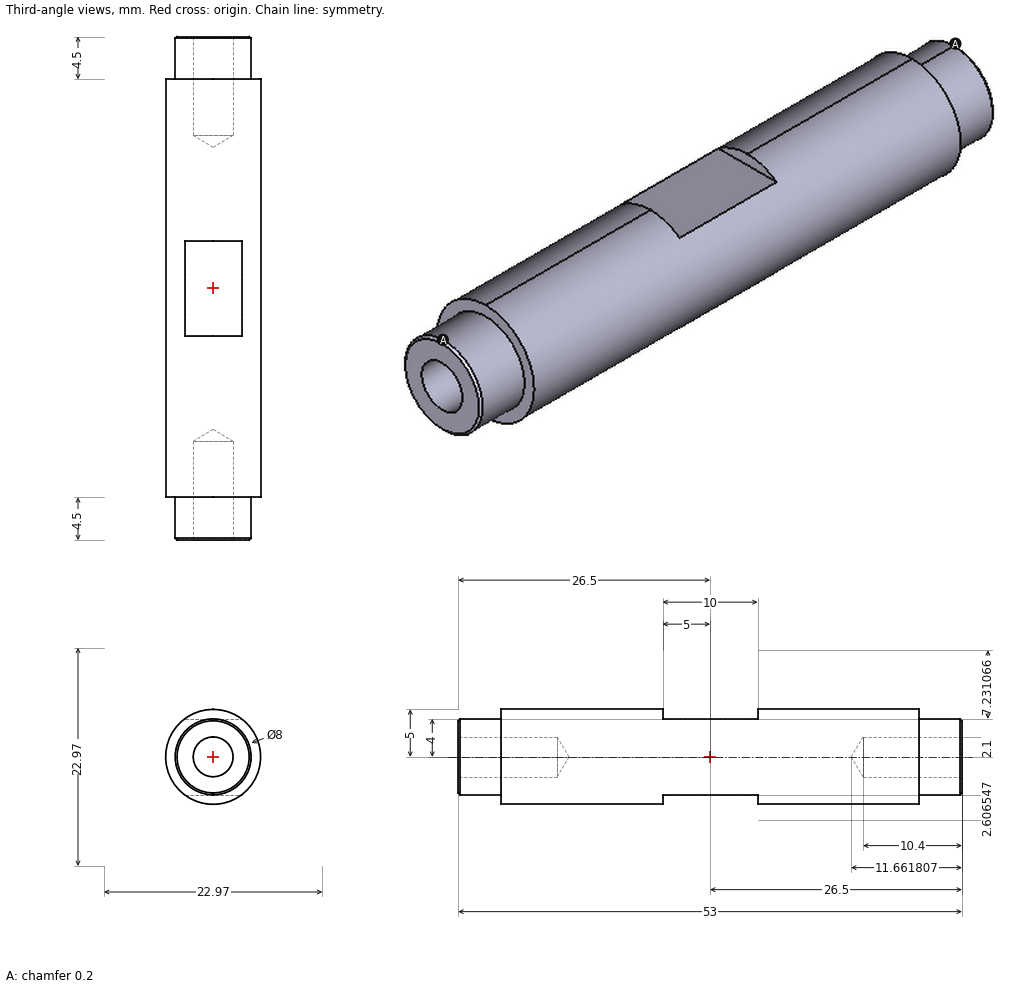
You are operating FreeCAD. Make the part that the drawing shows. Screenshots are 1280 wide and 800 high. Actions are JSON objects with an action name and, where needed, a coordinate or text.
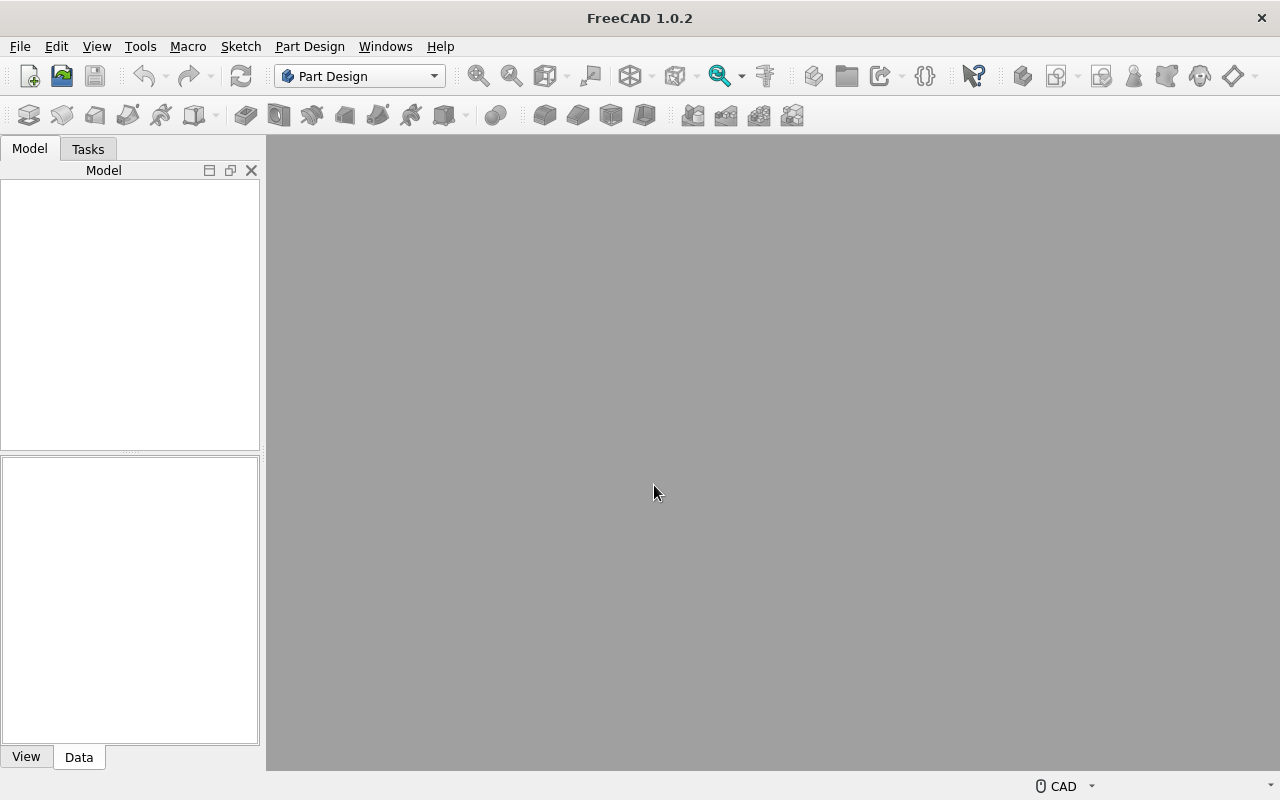
{"action": "left_click", "coordinate": [29, 76]}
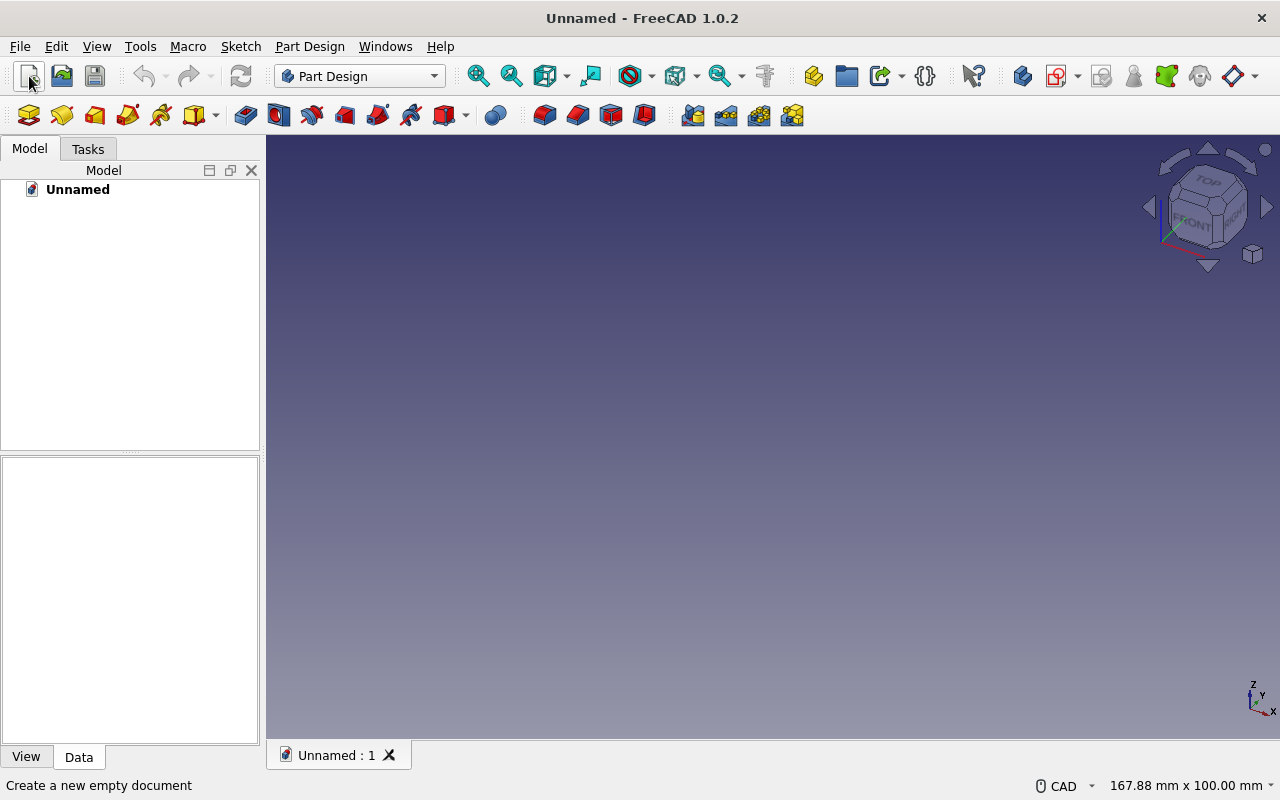
{"action": "left_click", "coordinate": [1056, 76]}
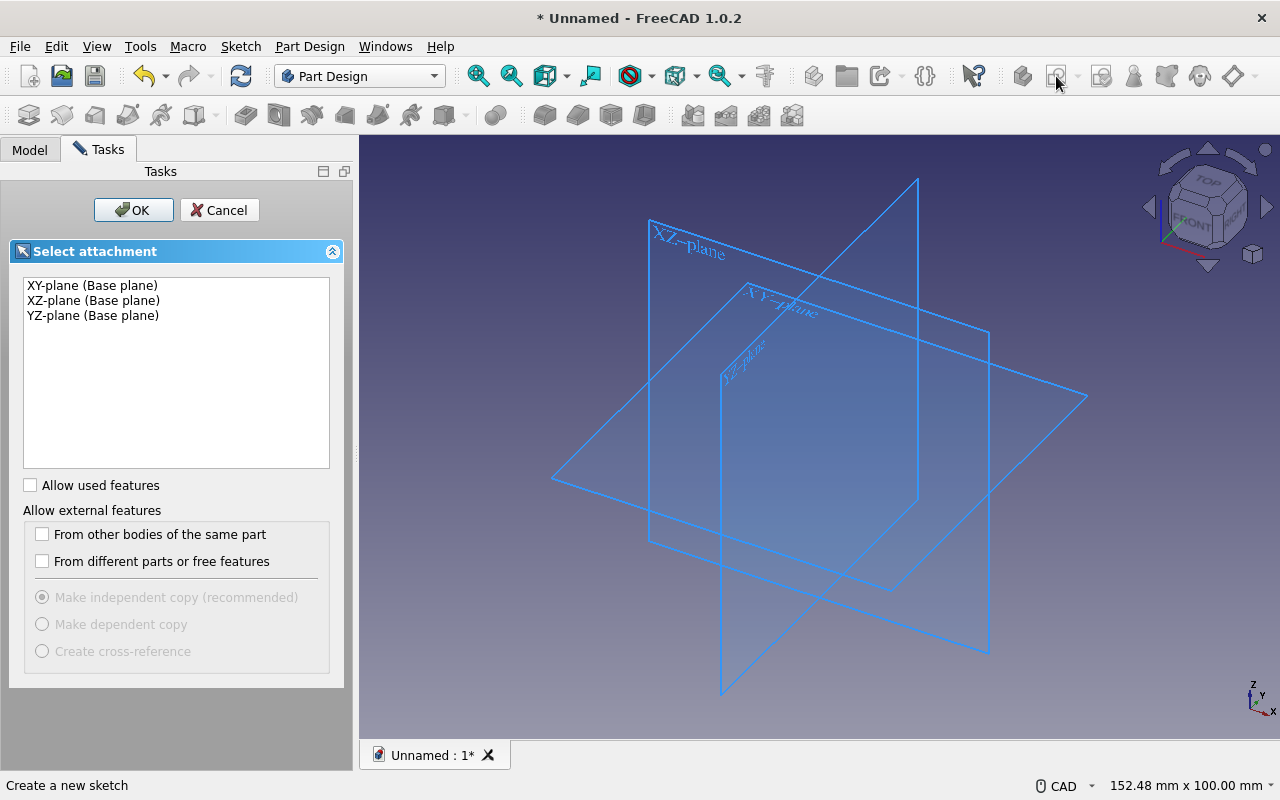
{"action": "left_click", "coordinate": [84, 316]}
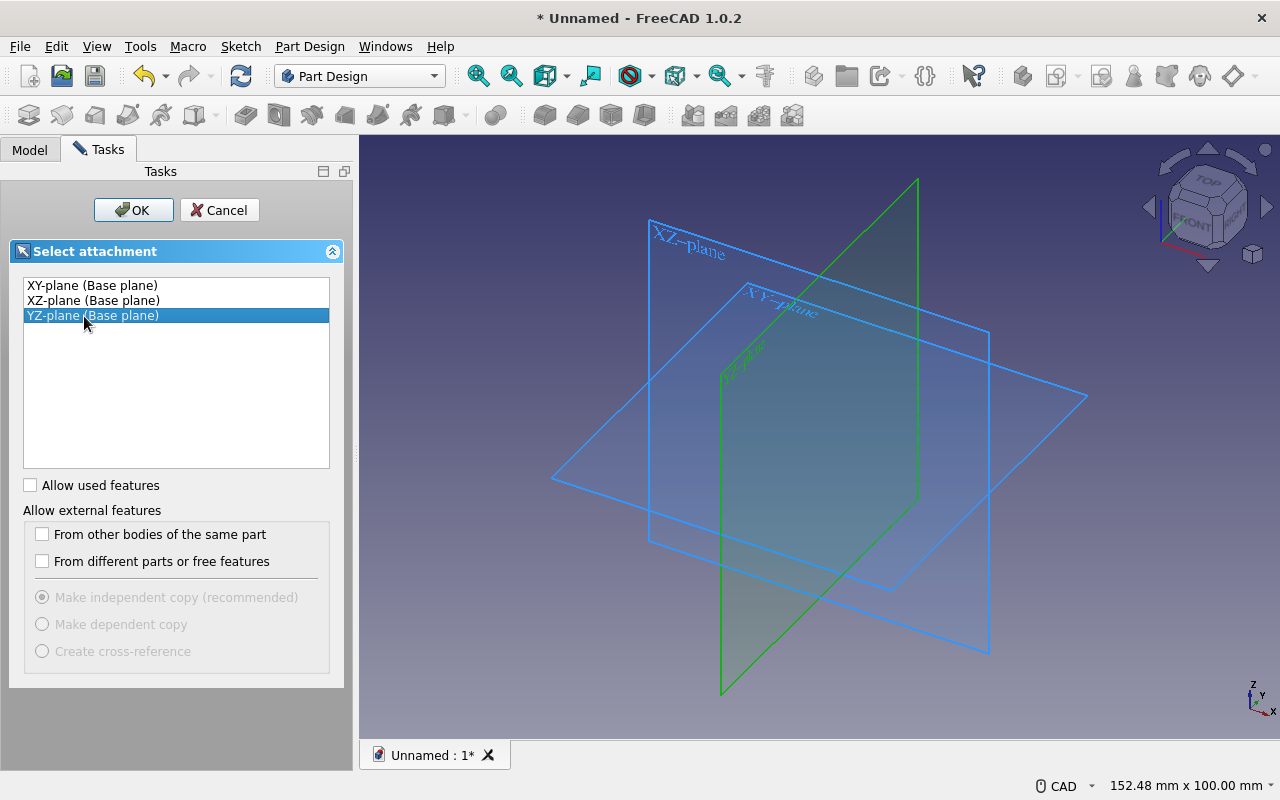
{"action": "left_click", "coordinate": [134, 210]}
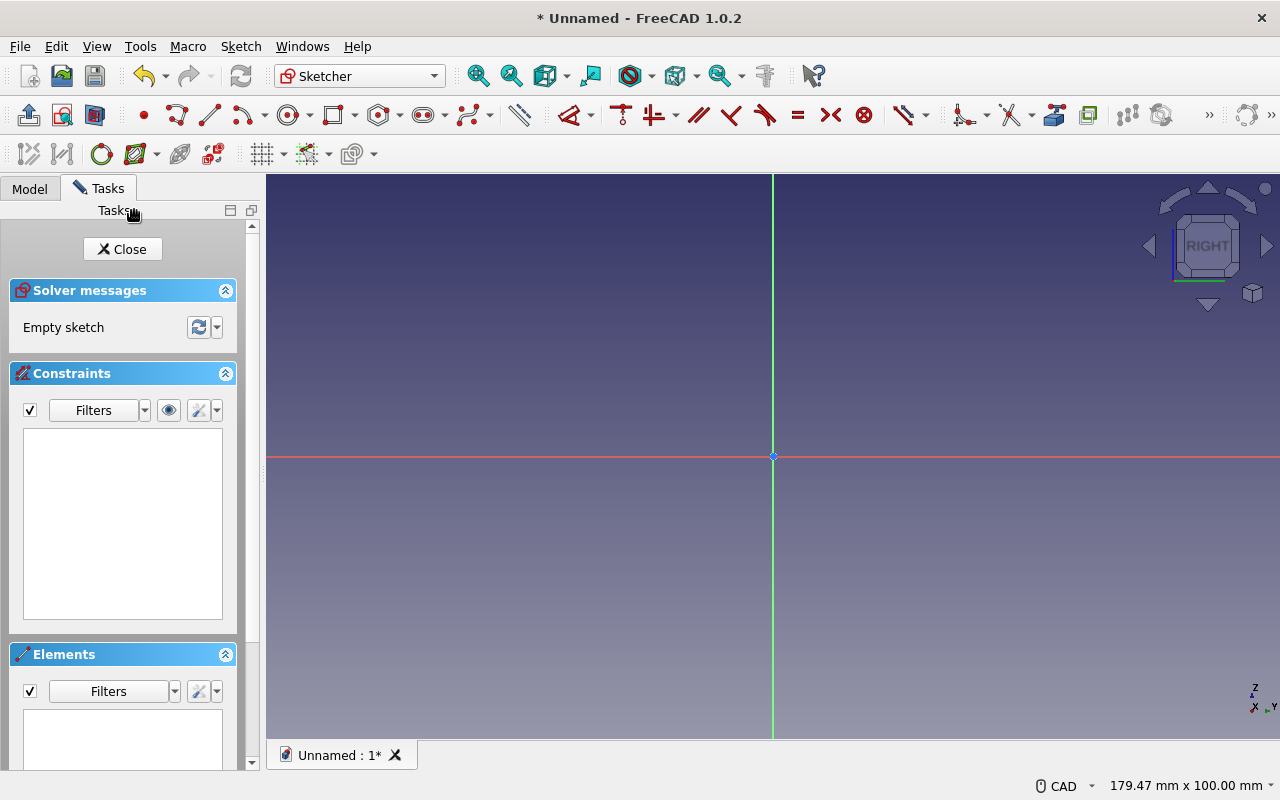
{"action": "scroll", "coordinate": [856, 425], "scroll_direction": "up", "scroll_amount": 3}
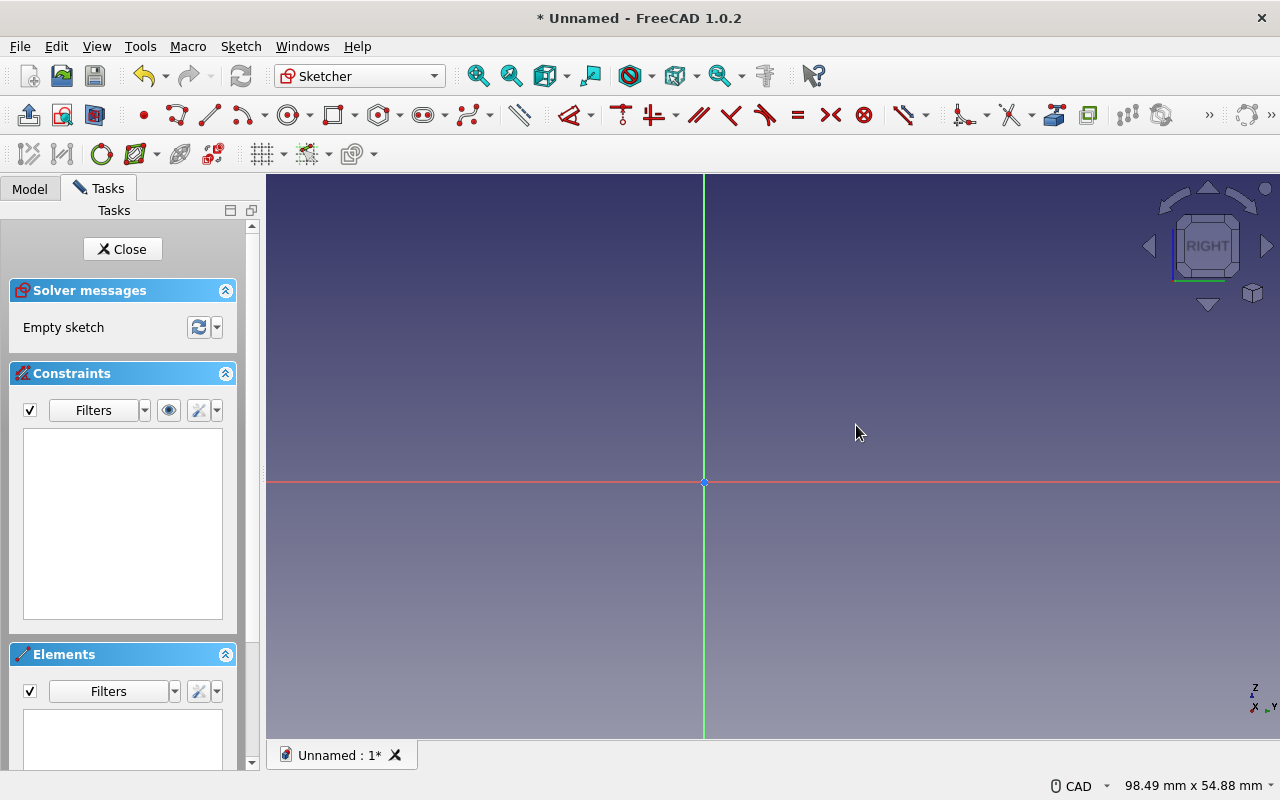
{"action": "left_click", "coordinate": [332, 116]}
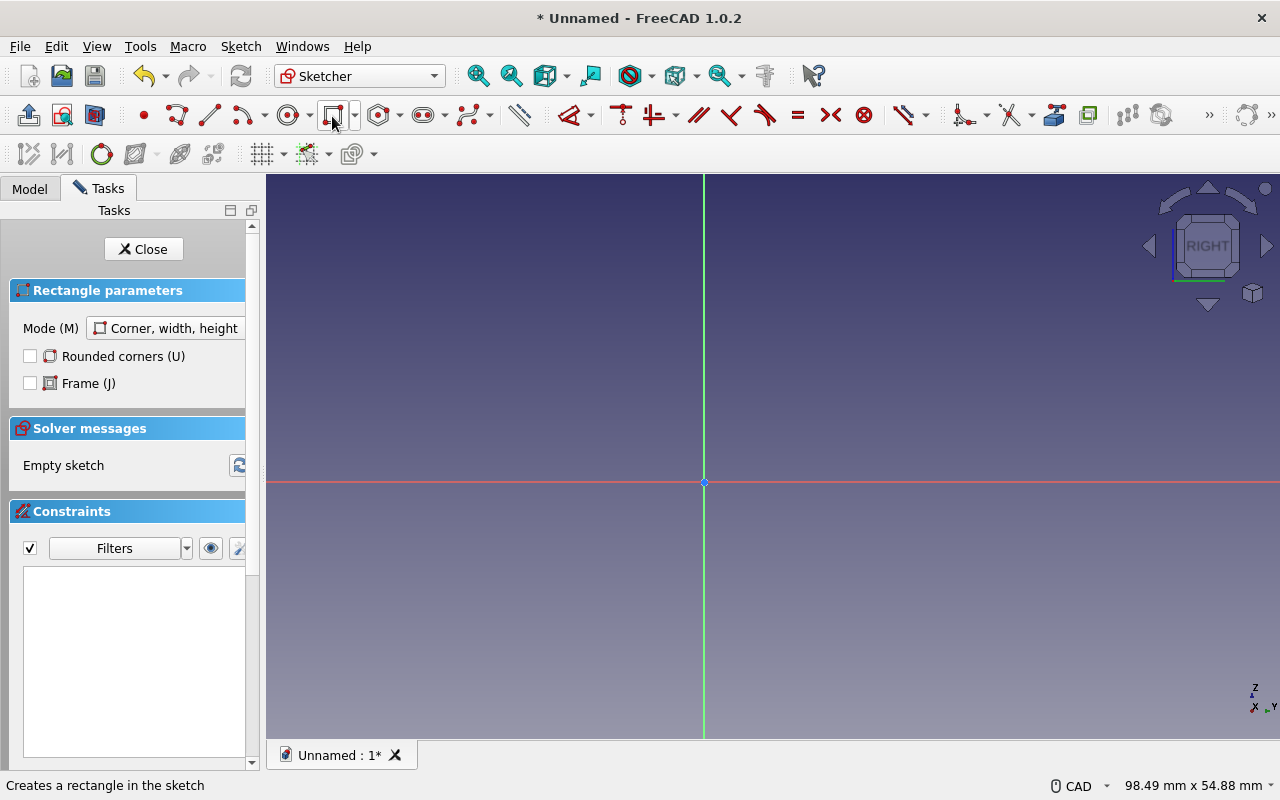
{"action": "left_click", "coordinate": [431, 431]}
{"action": "left_click", "coordinate": [977, 482]}
{"action": "key", "text": "Escape"}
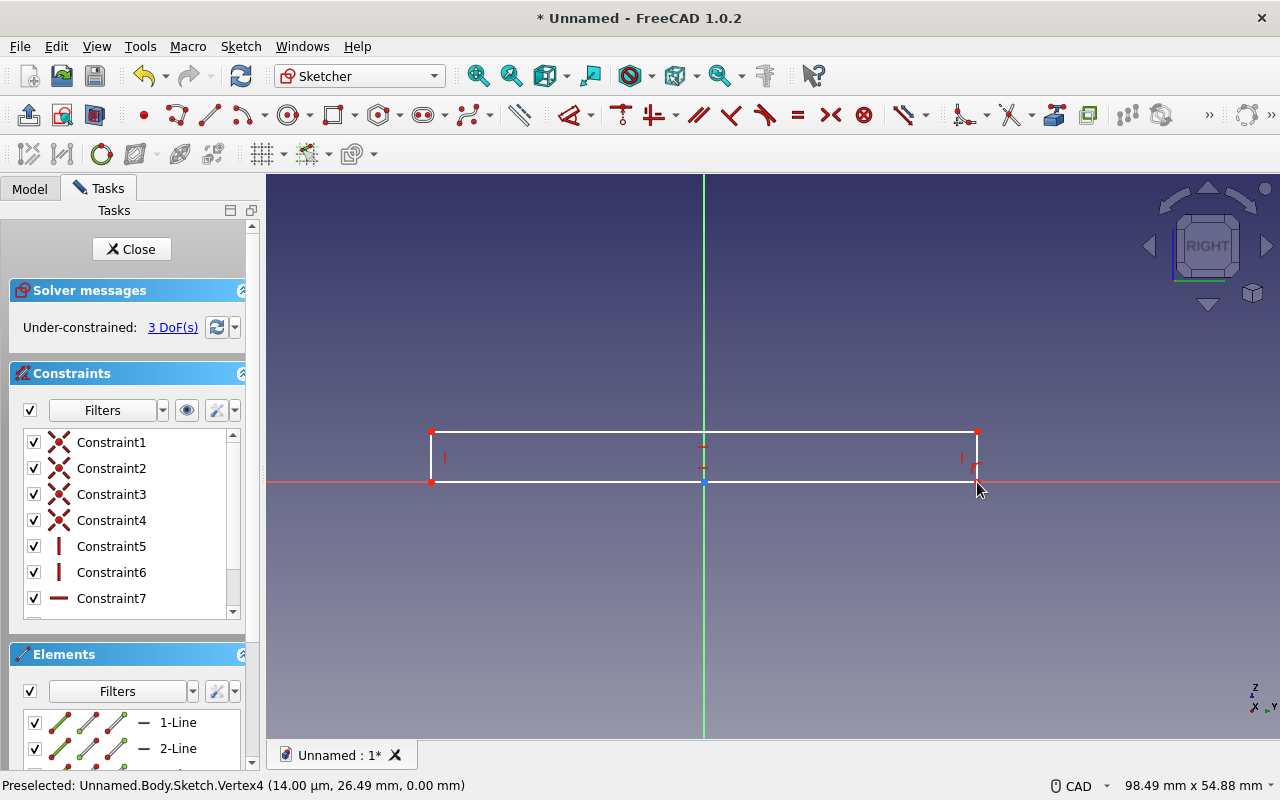
{"action": "left_click", "coordinate": [568, 116]}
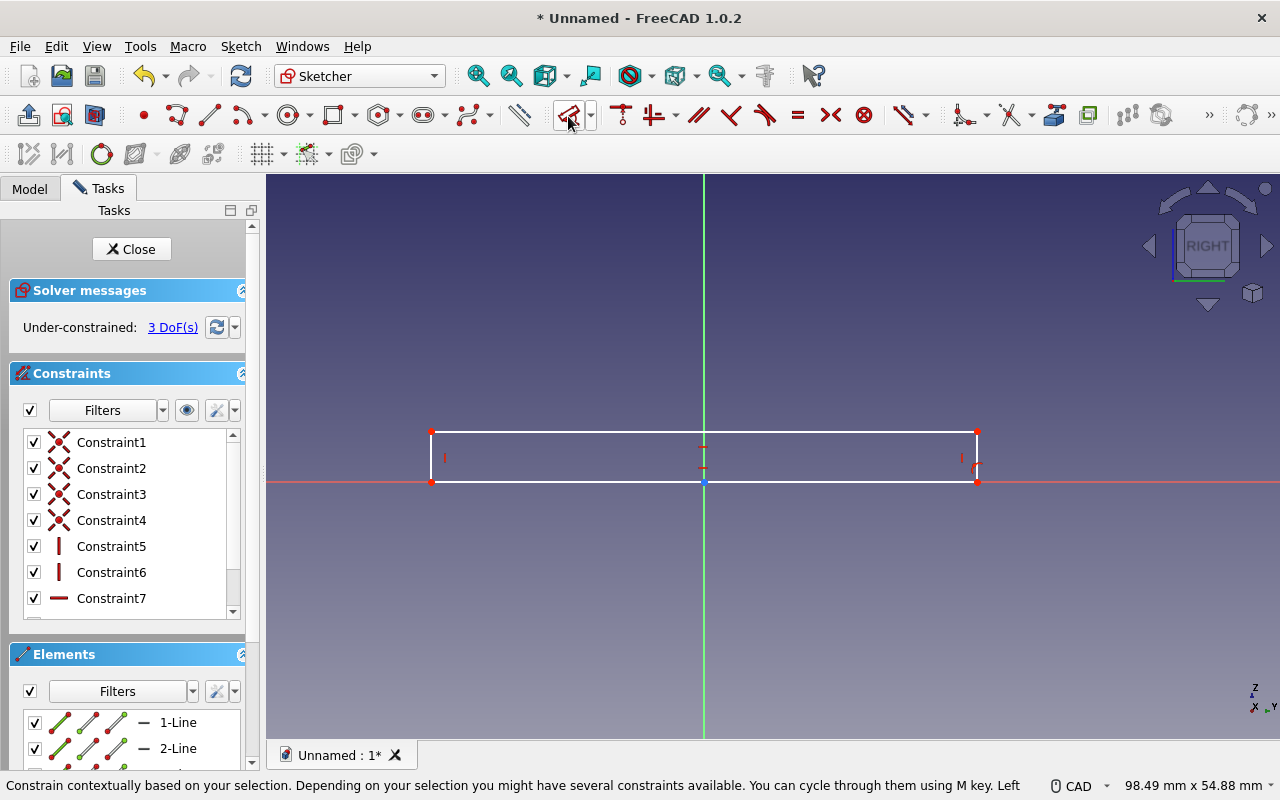
{"action": "left_click", "coordinate": [431, 447]}
{"action": "left_click", "coordinate": [397, 457]}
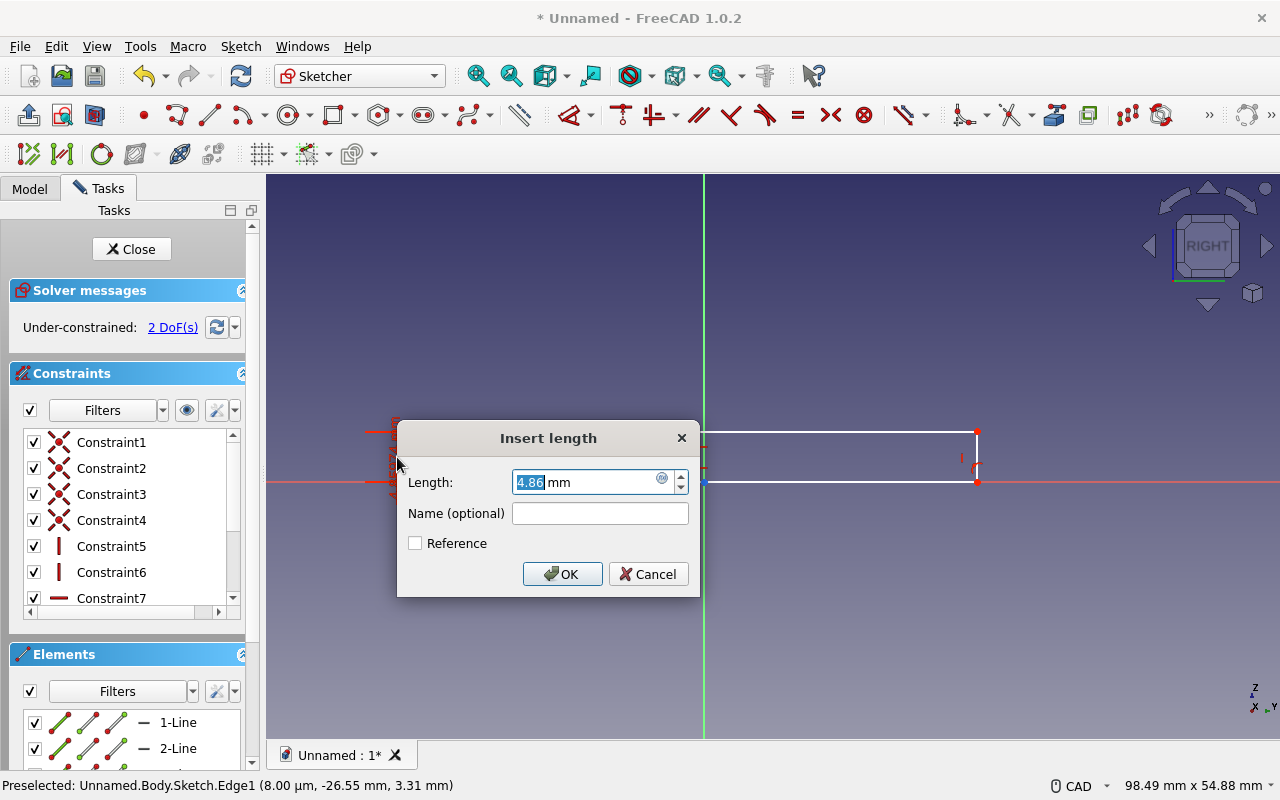
{"action": "type", "text": "5"}
{"action": "key", "text": "Return"}